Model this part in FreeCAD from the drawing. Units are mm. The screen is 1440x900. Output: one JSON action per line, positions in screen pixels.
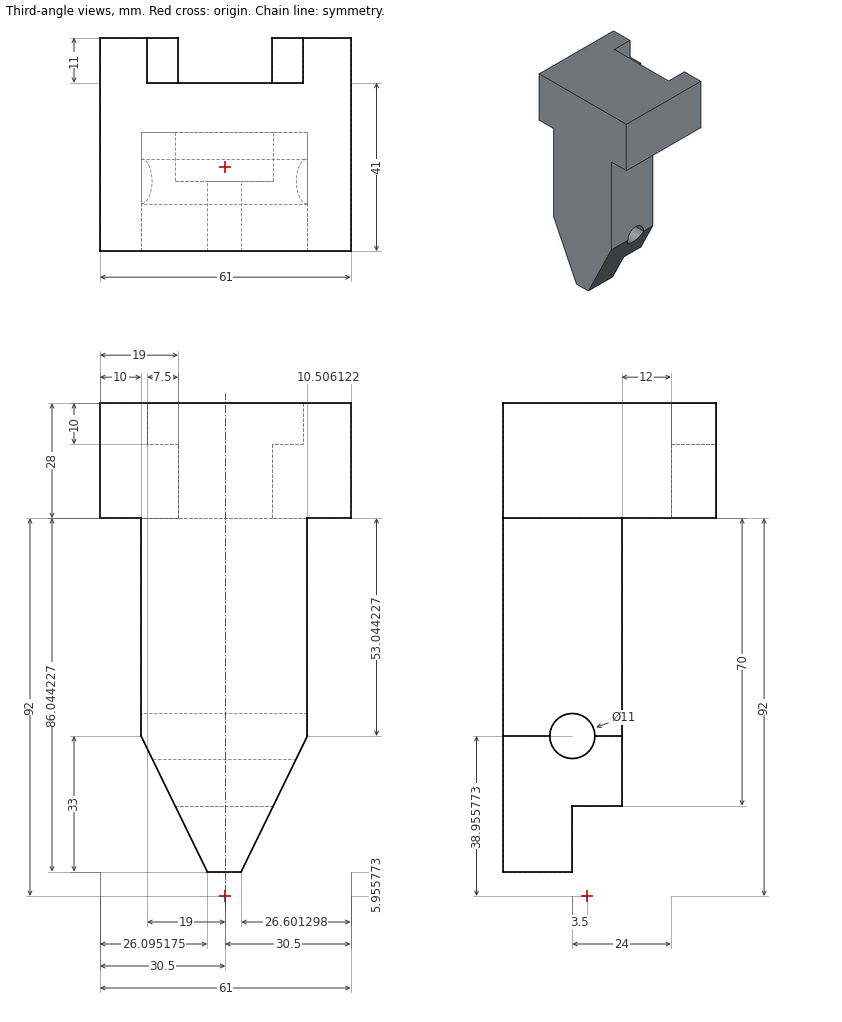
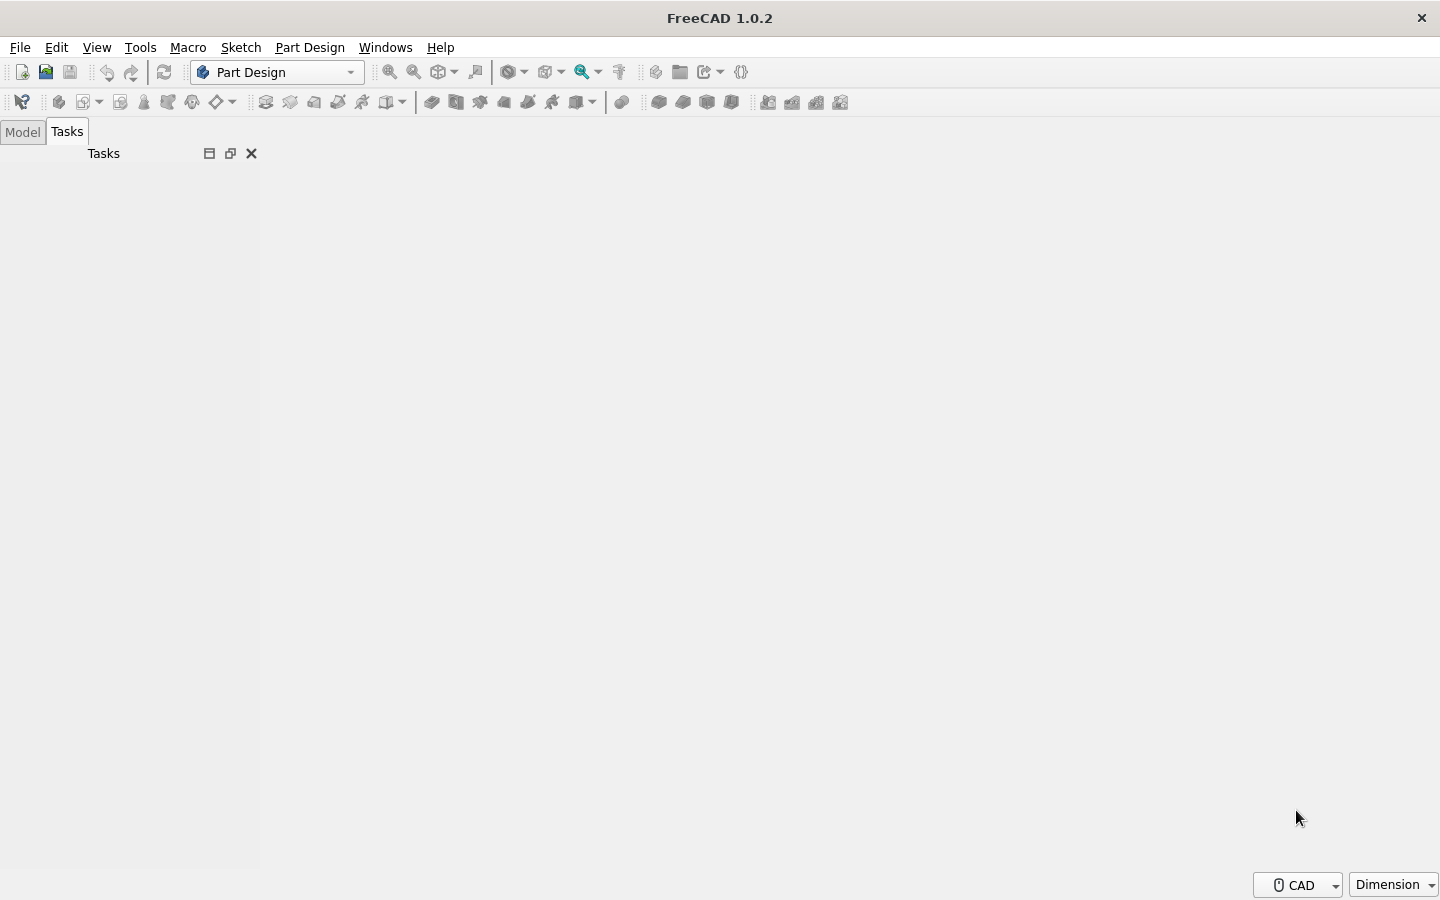
{"action": "left_click", "coordinate": [22, 72]}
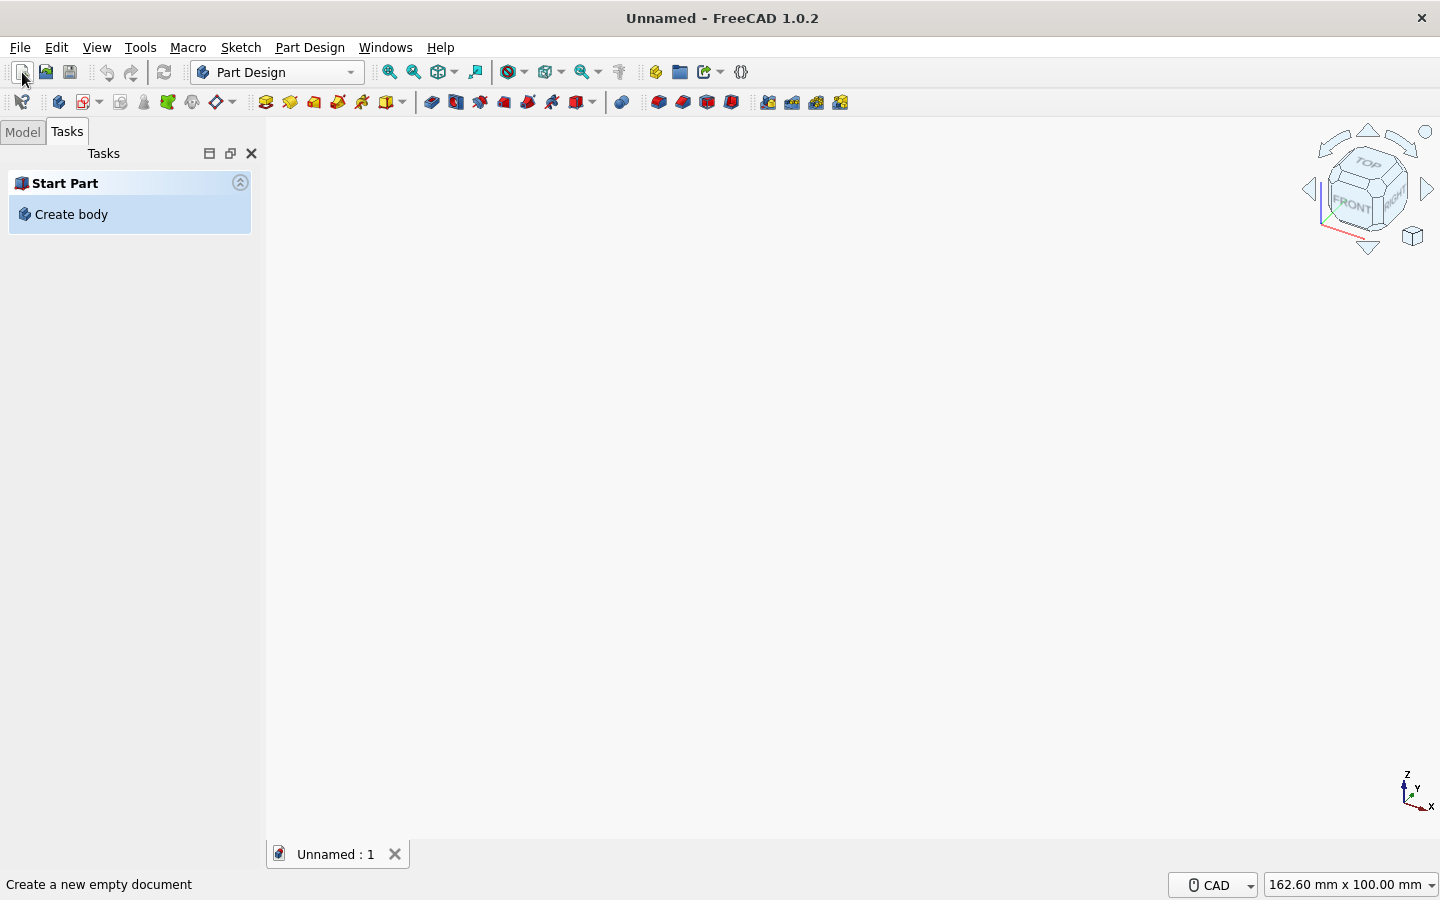
{"action": "left_click", "coordinate": [84, 102]}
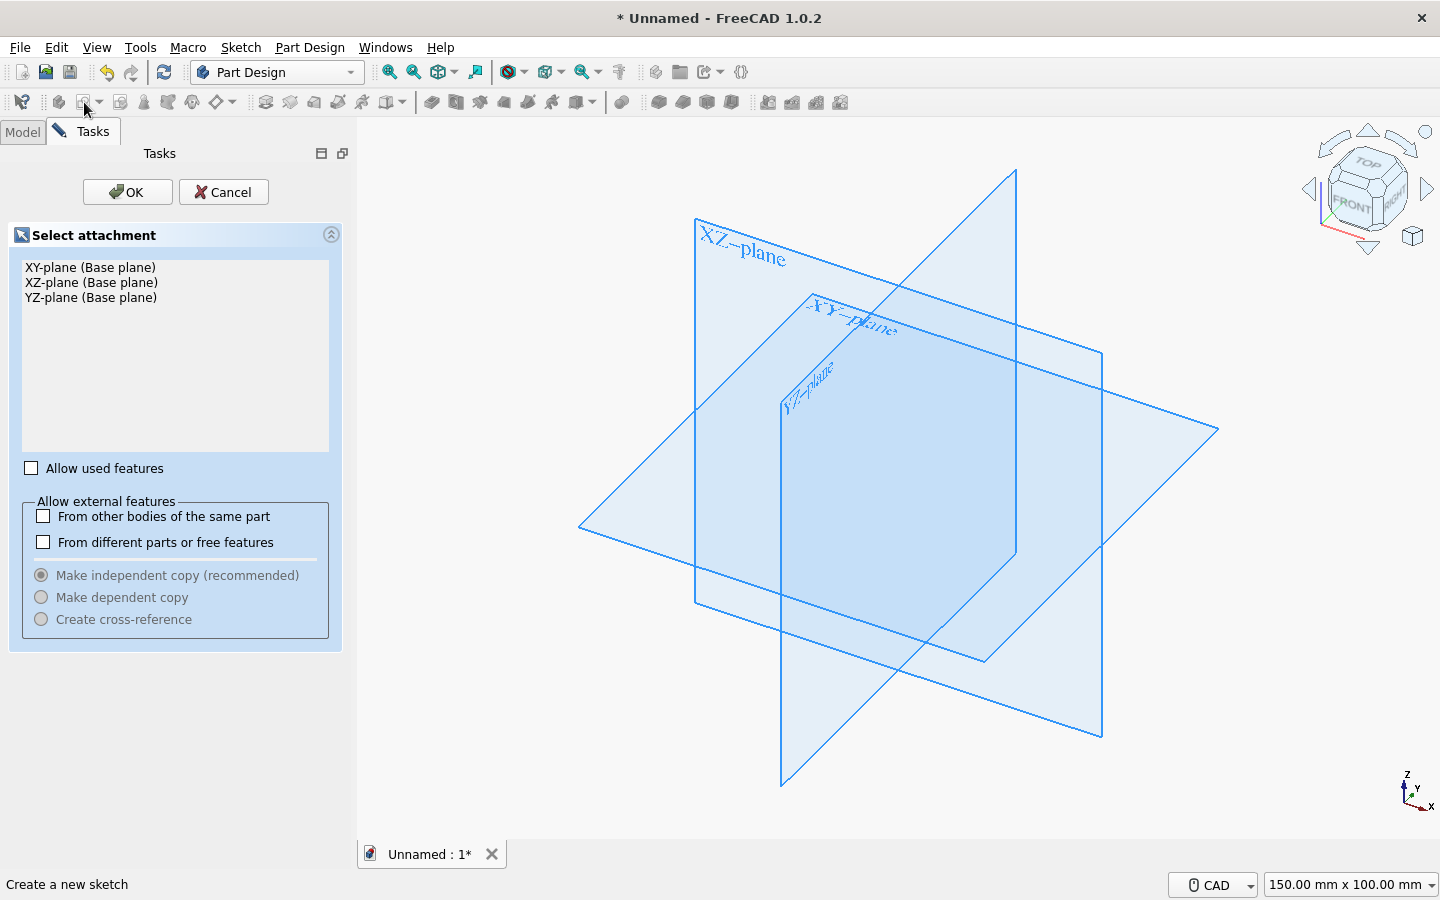
{"action": "left_click", "coordinate": [82, 268]}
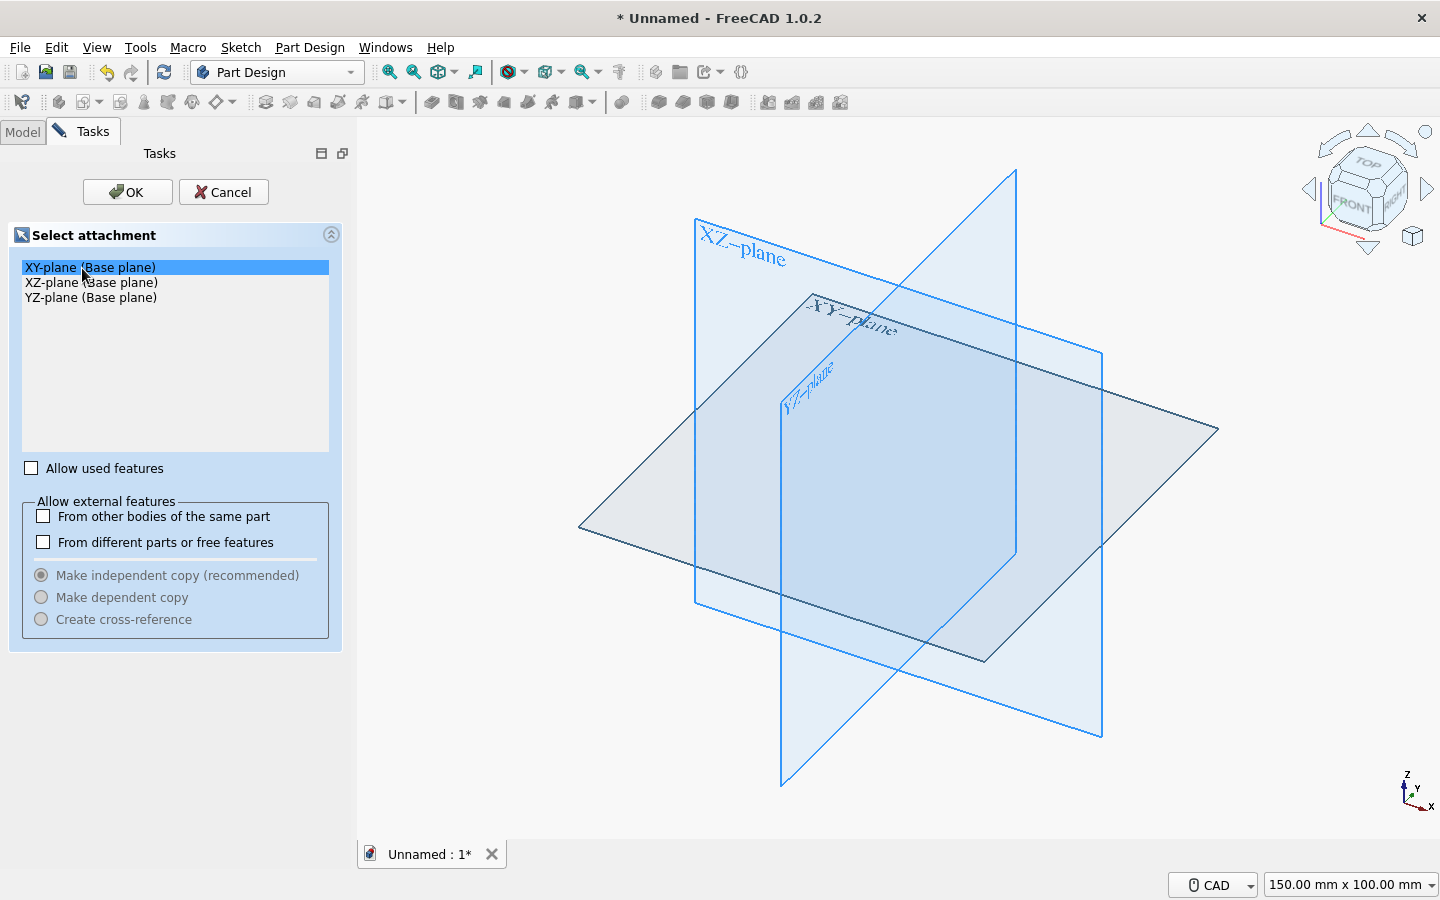
{"action": "left_click", "coordinate": [128, 192]}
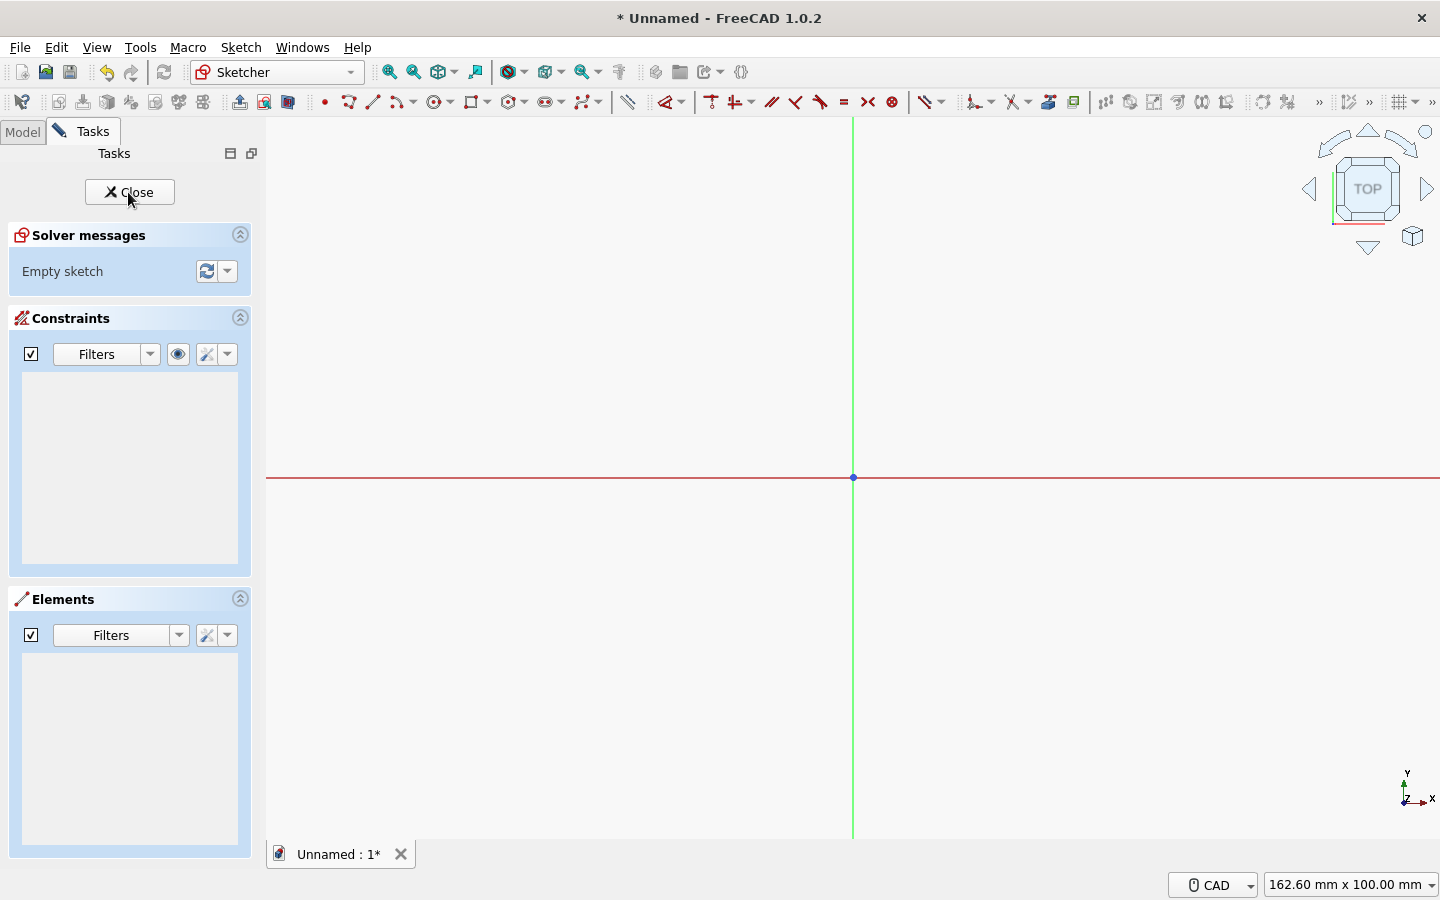
{"action": "scroll", "coordinate": [992, 478], "scroll_direction": "up", "scroll_amount": 2}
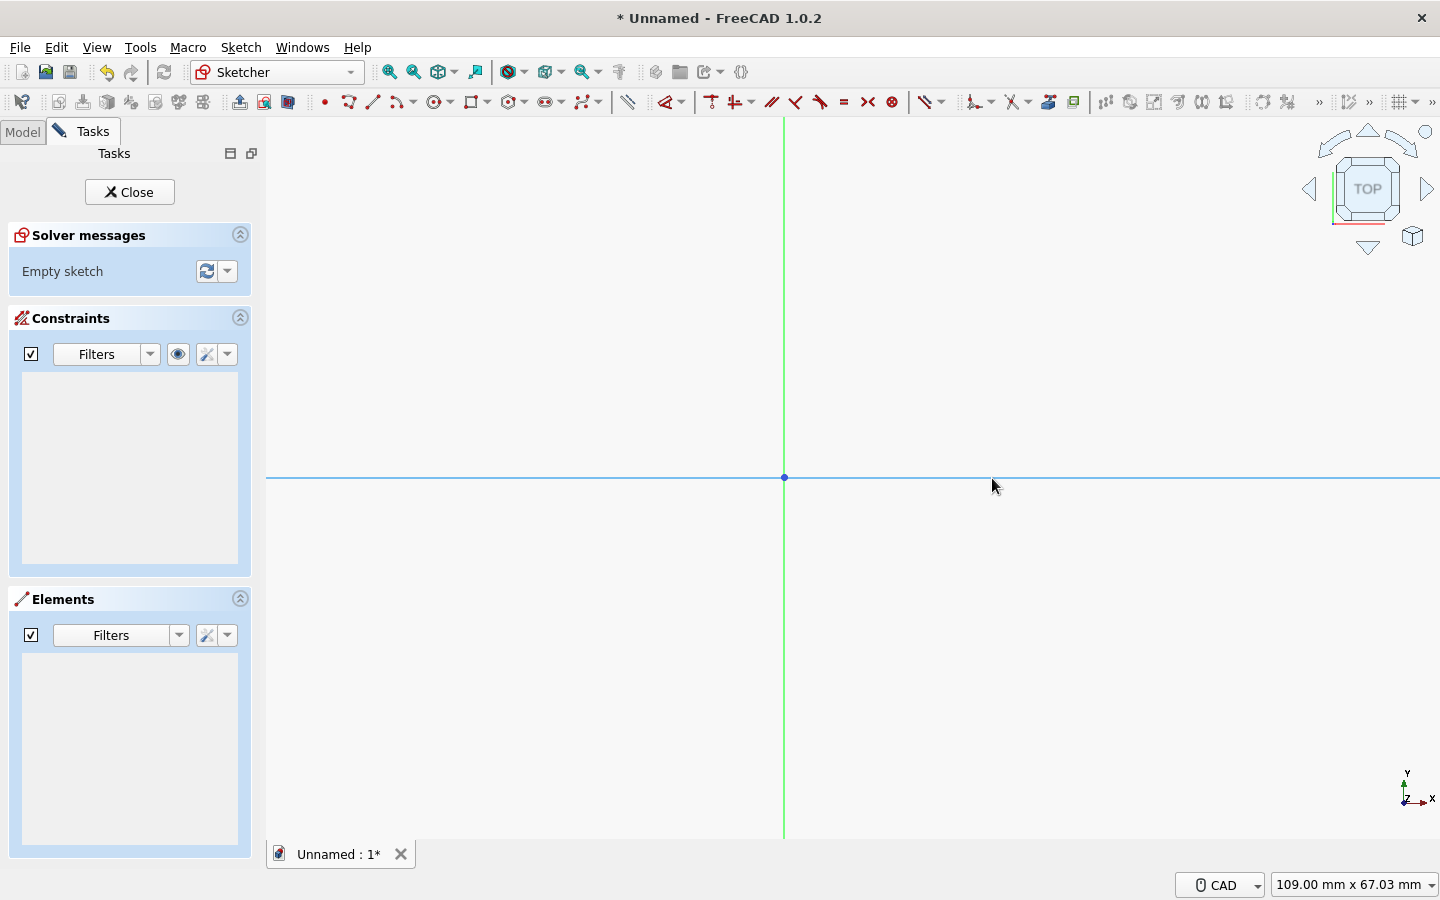
{"action": "key", "text": "g v"}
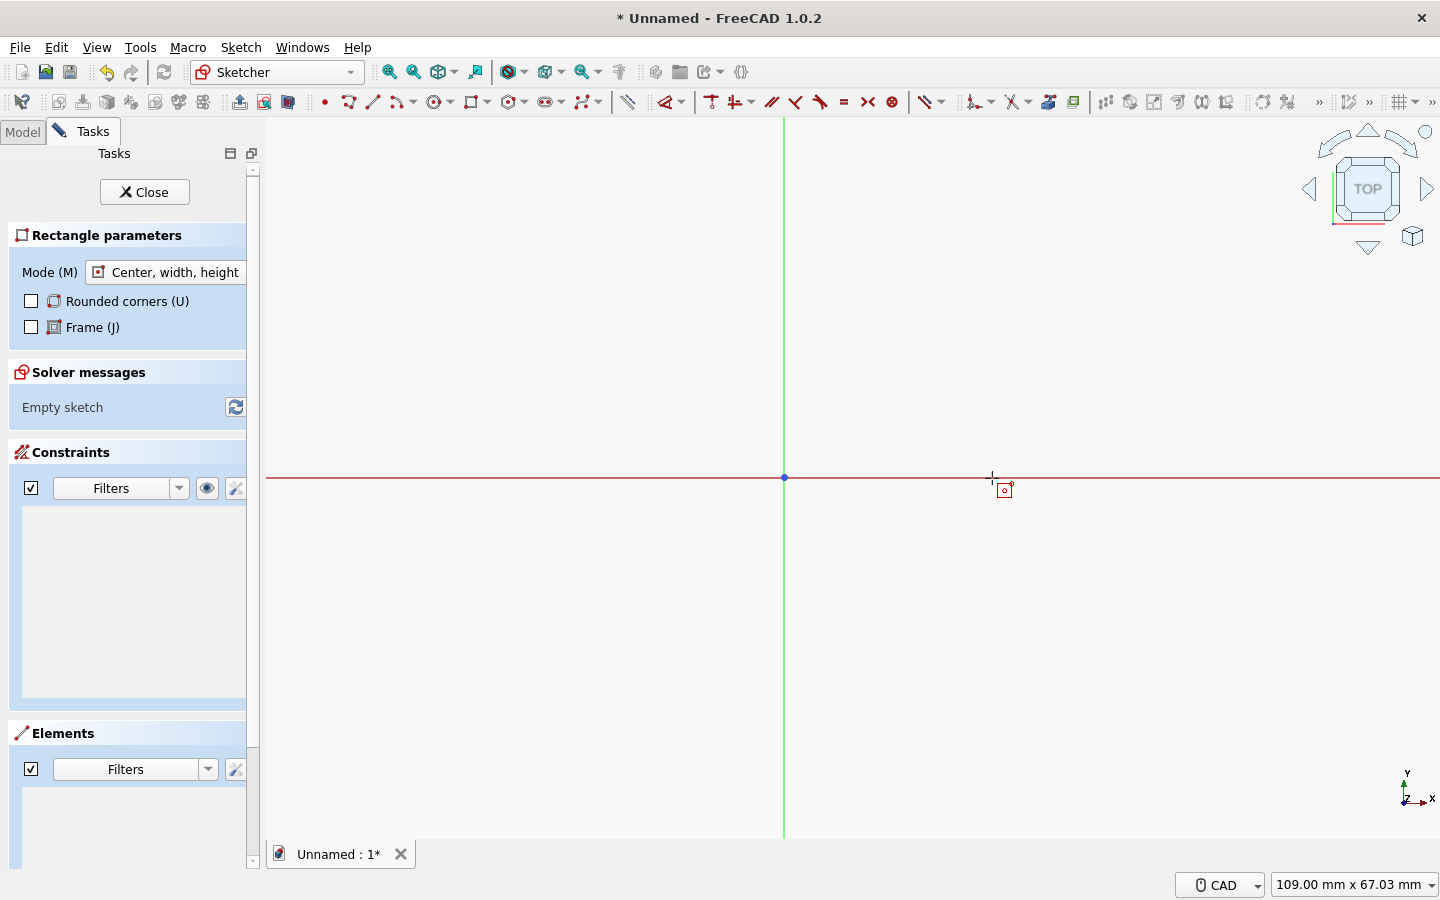
{"action": "left_click", "coordinate": [784, 478]}
{"action": "left_click", "coordinate": [1113, 257]}
{"action": "key", "text": "Escape"}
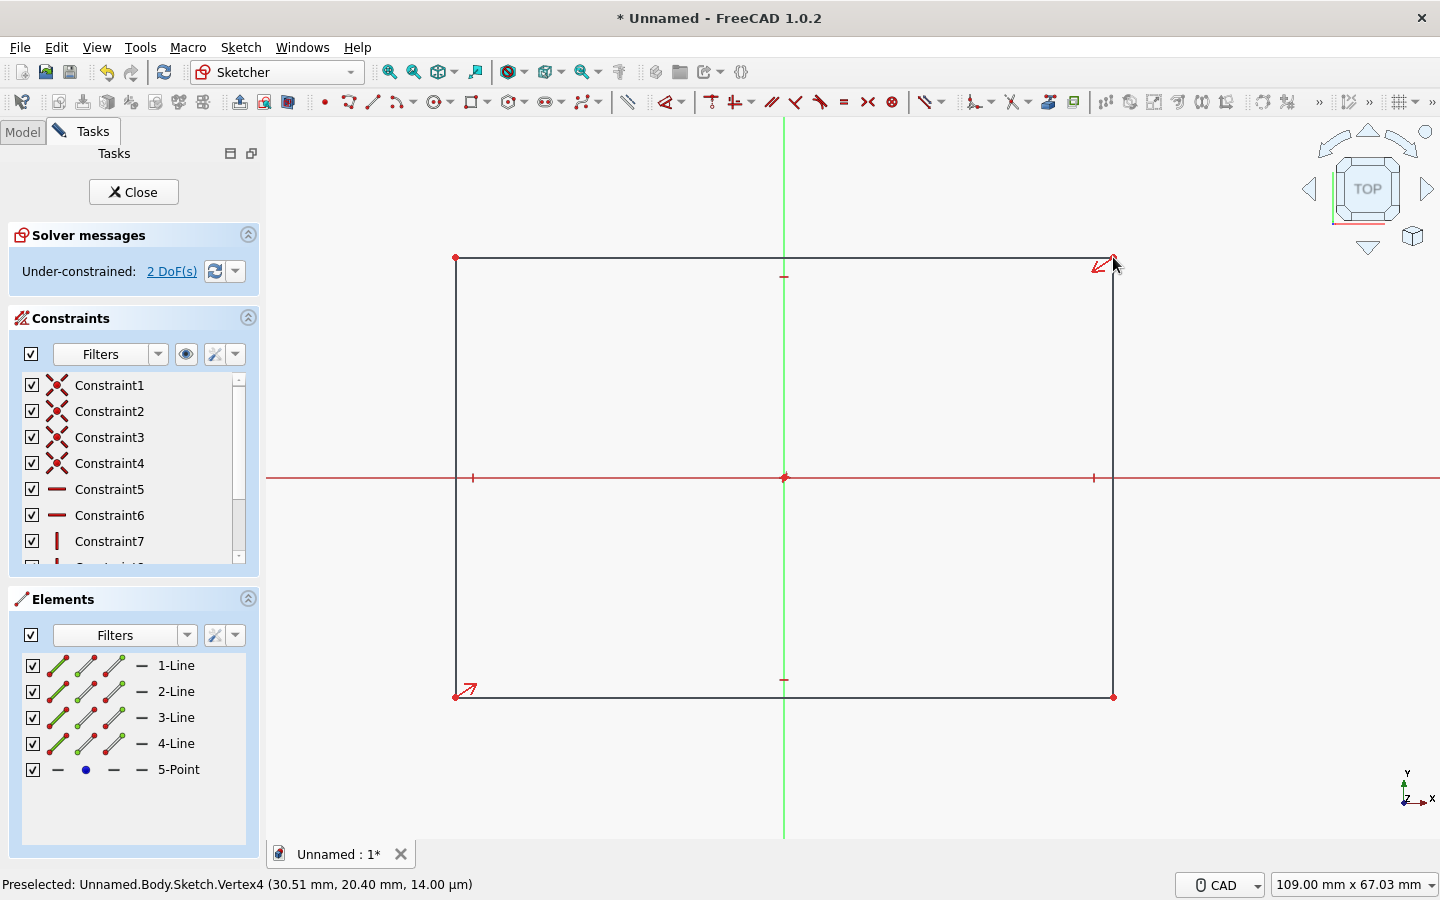
{"action": "left_click", "coordinate": [666, 102]}